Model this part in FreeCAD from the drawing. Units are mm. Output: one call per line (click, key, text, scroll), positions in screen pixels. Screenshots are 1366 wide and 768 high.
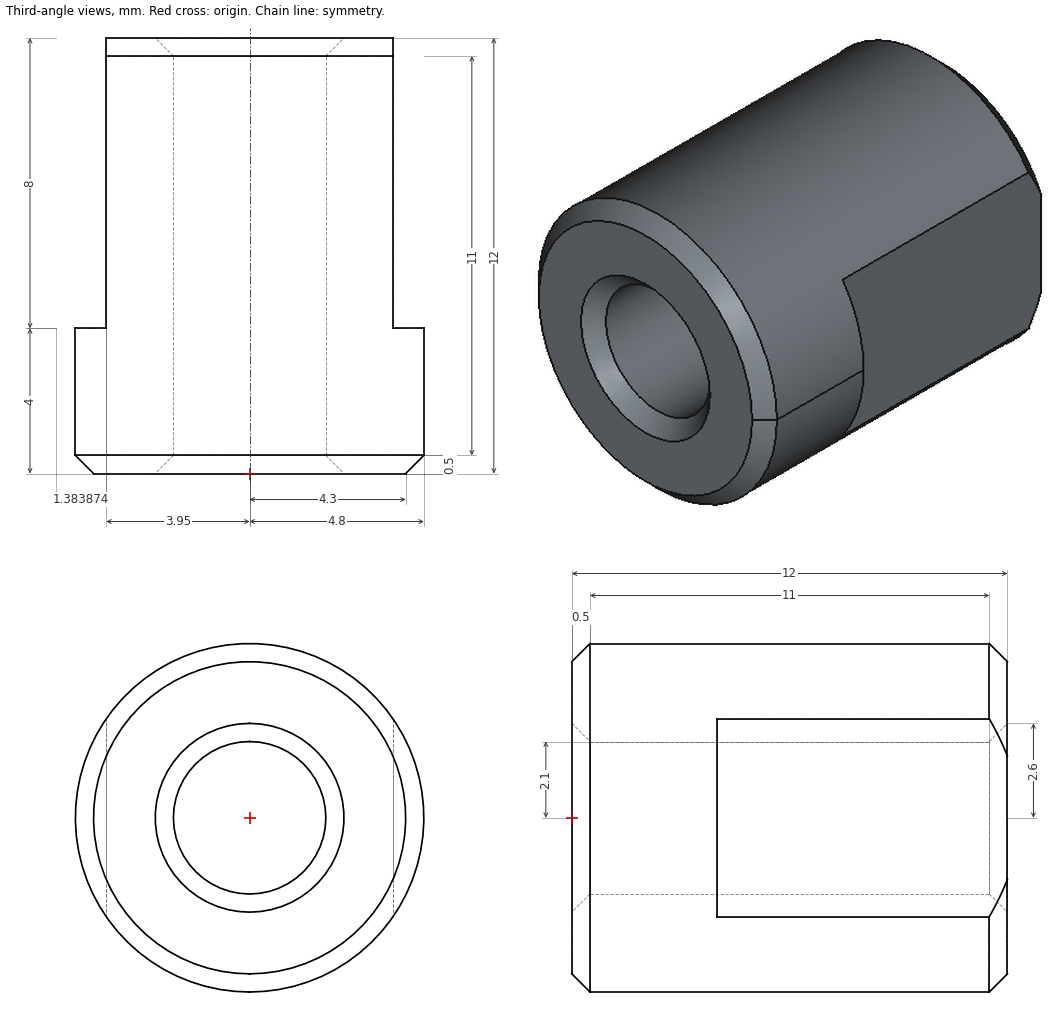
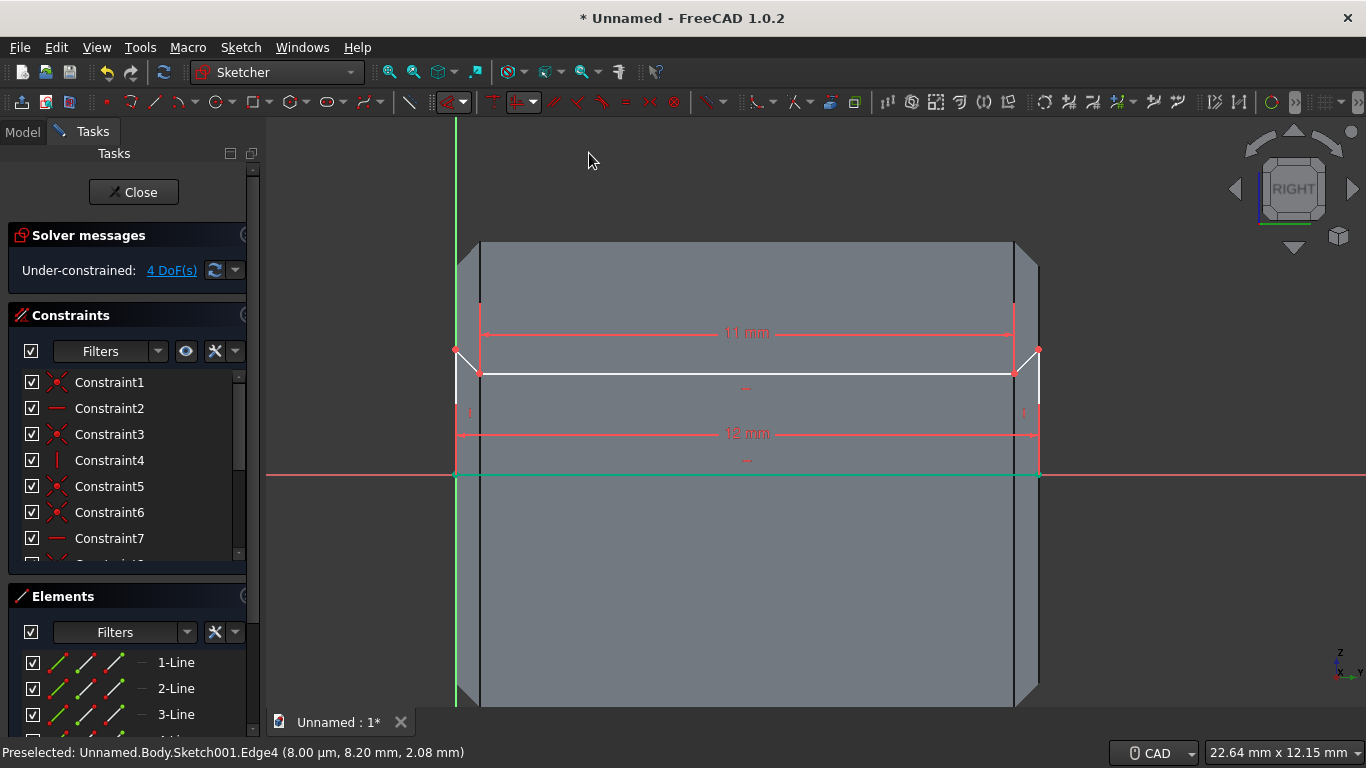
click(1039, 437)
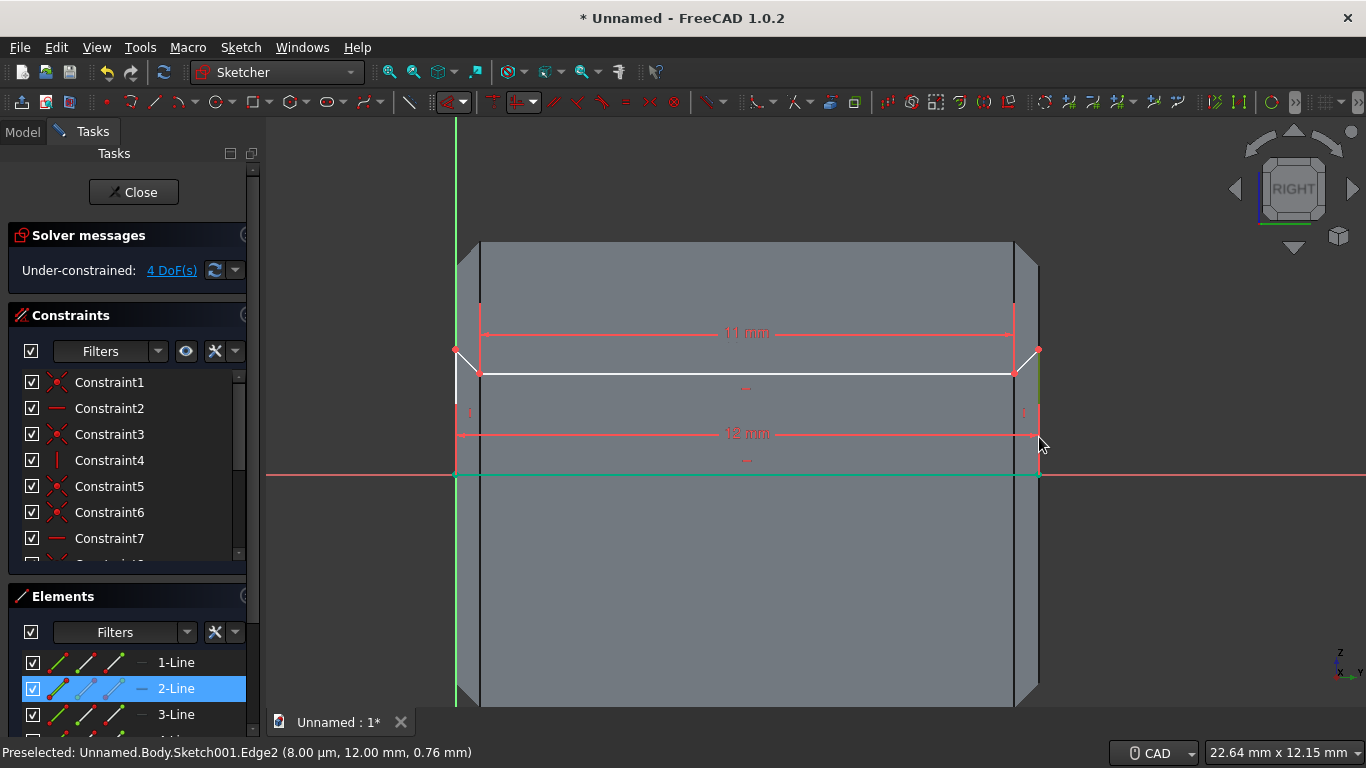
key(i)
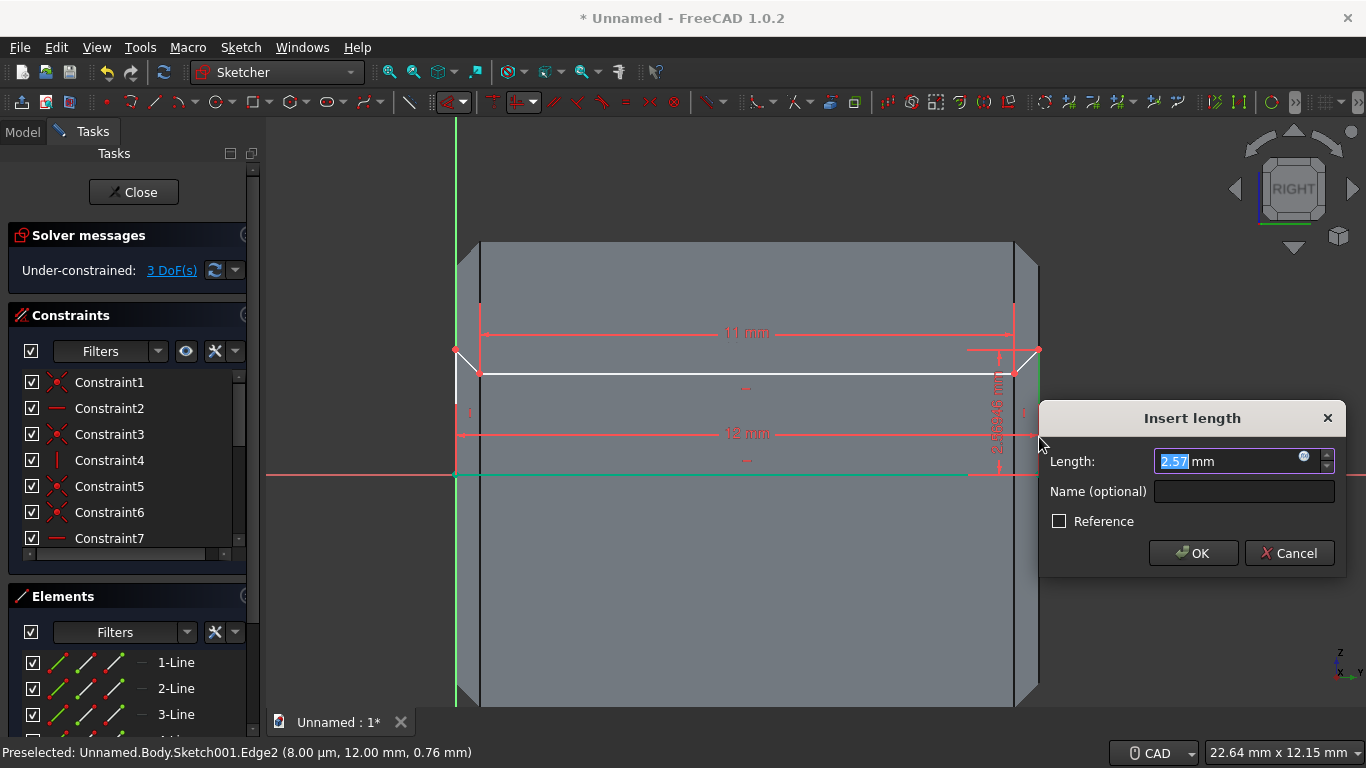
text(2.6)
key(Return)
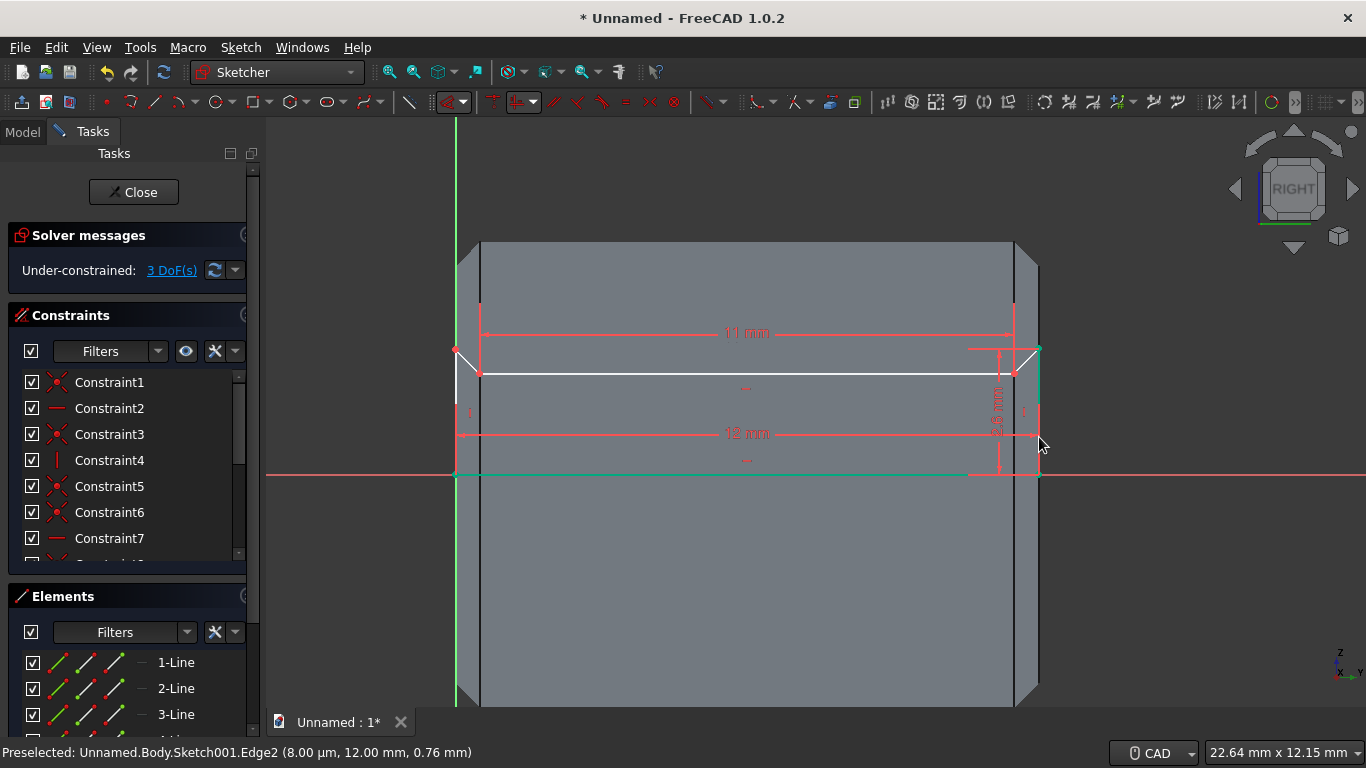
click(456, 387)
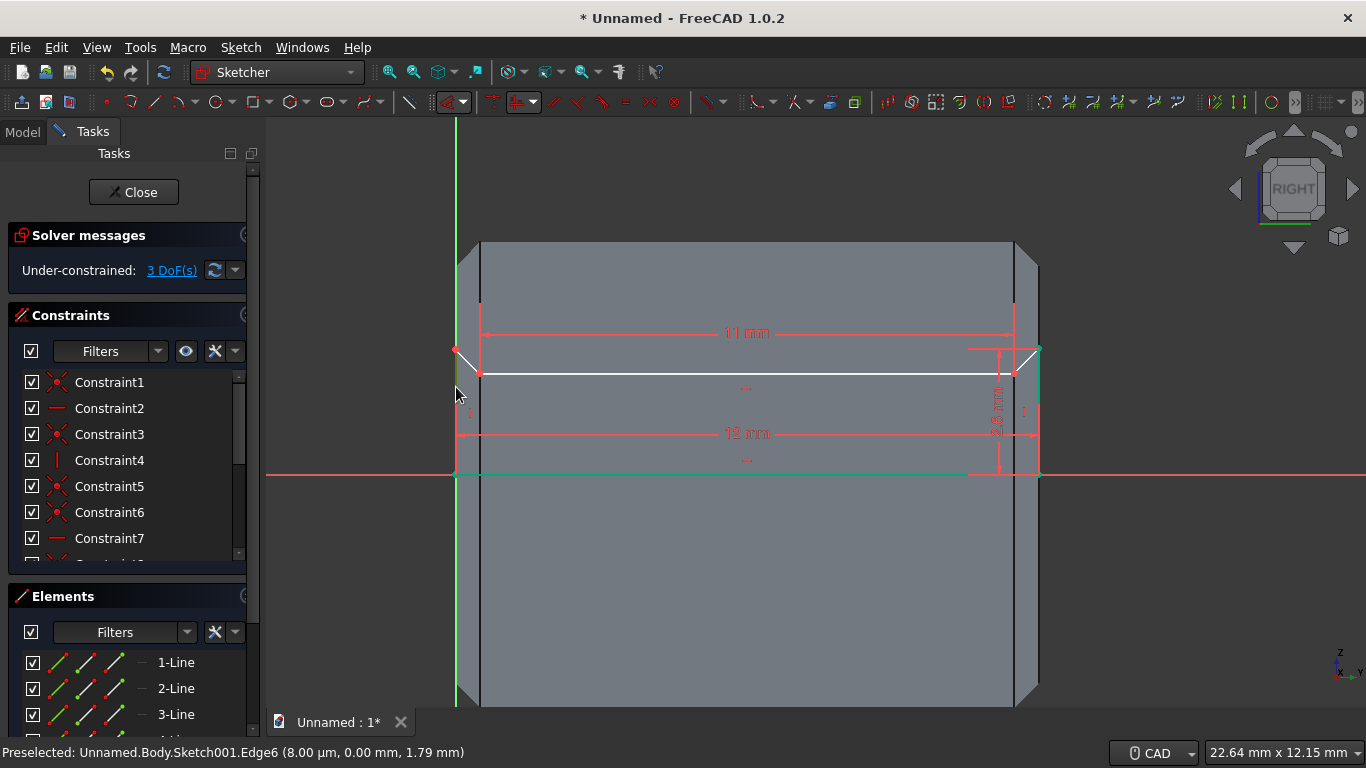
click(466, 102)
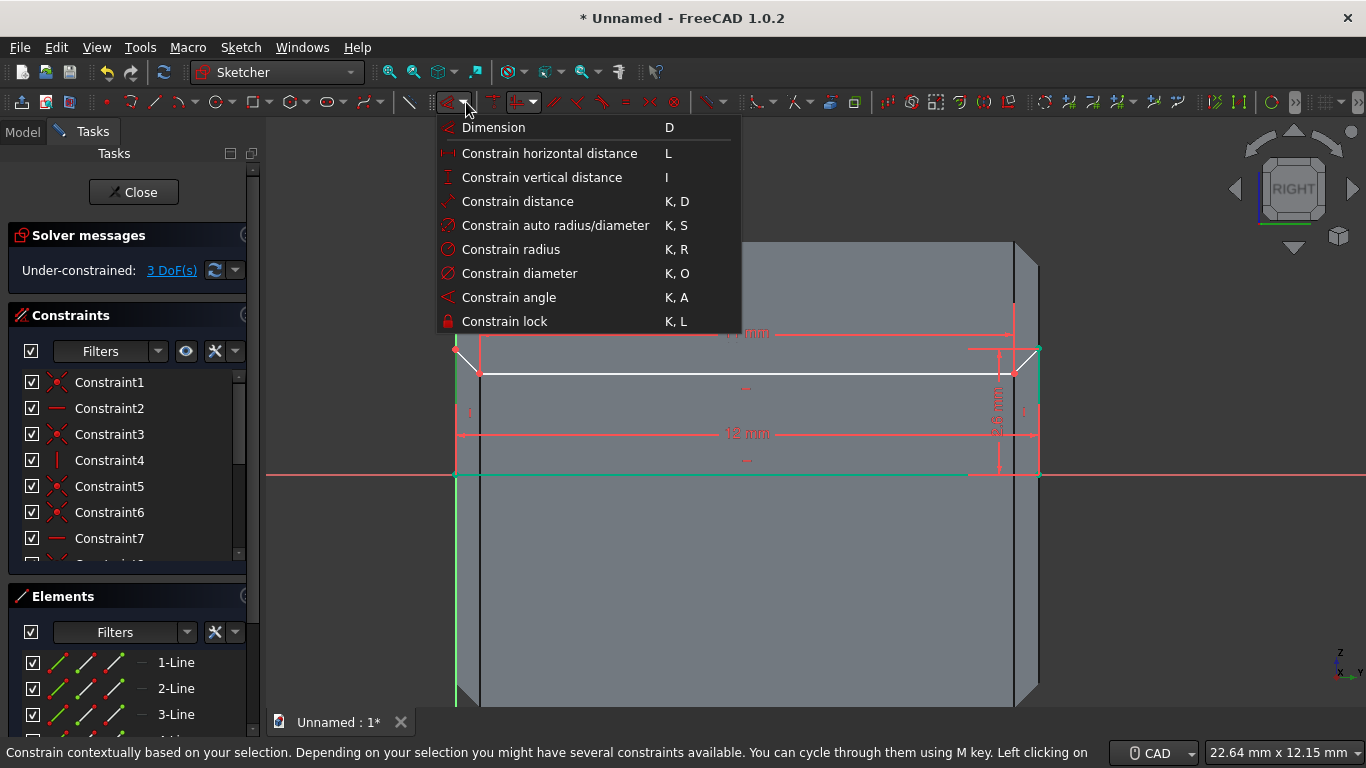
click(589, 177)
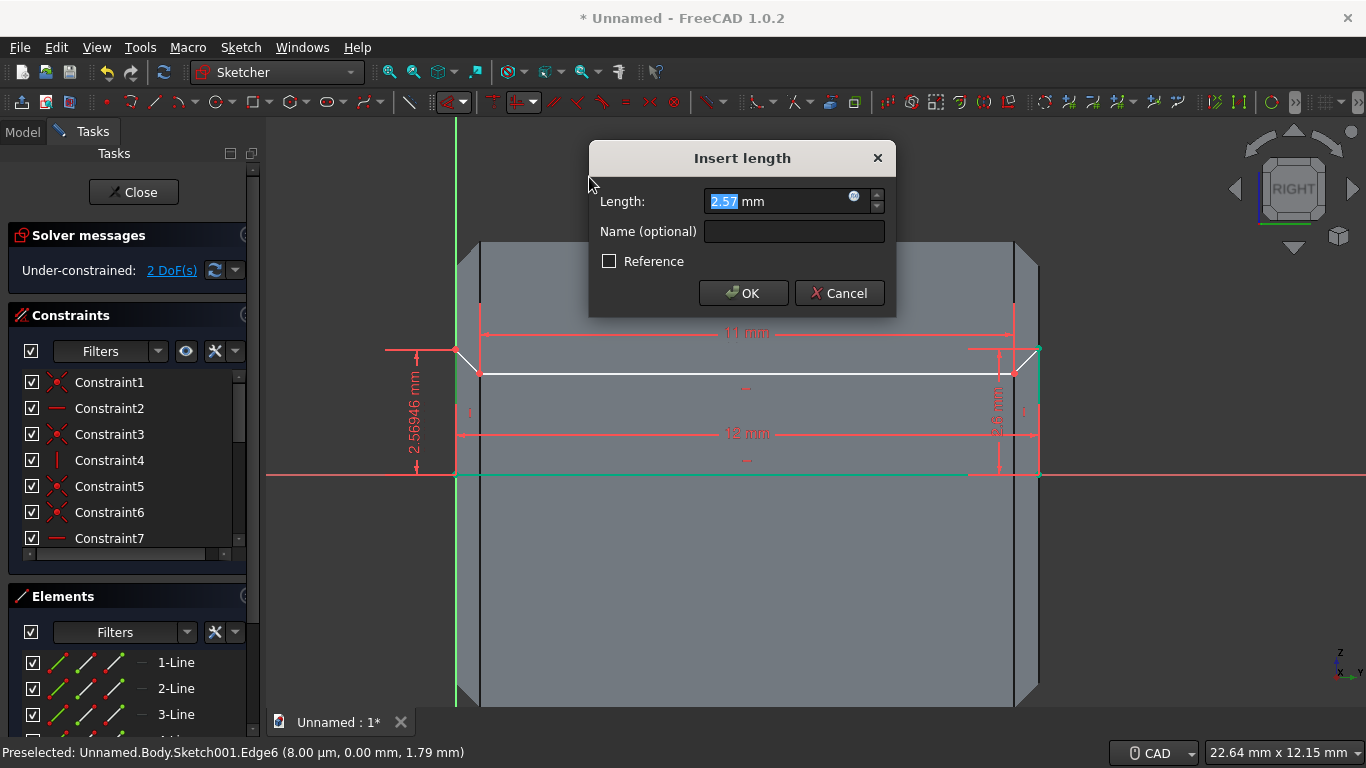
text(2.6)
key(Return)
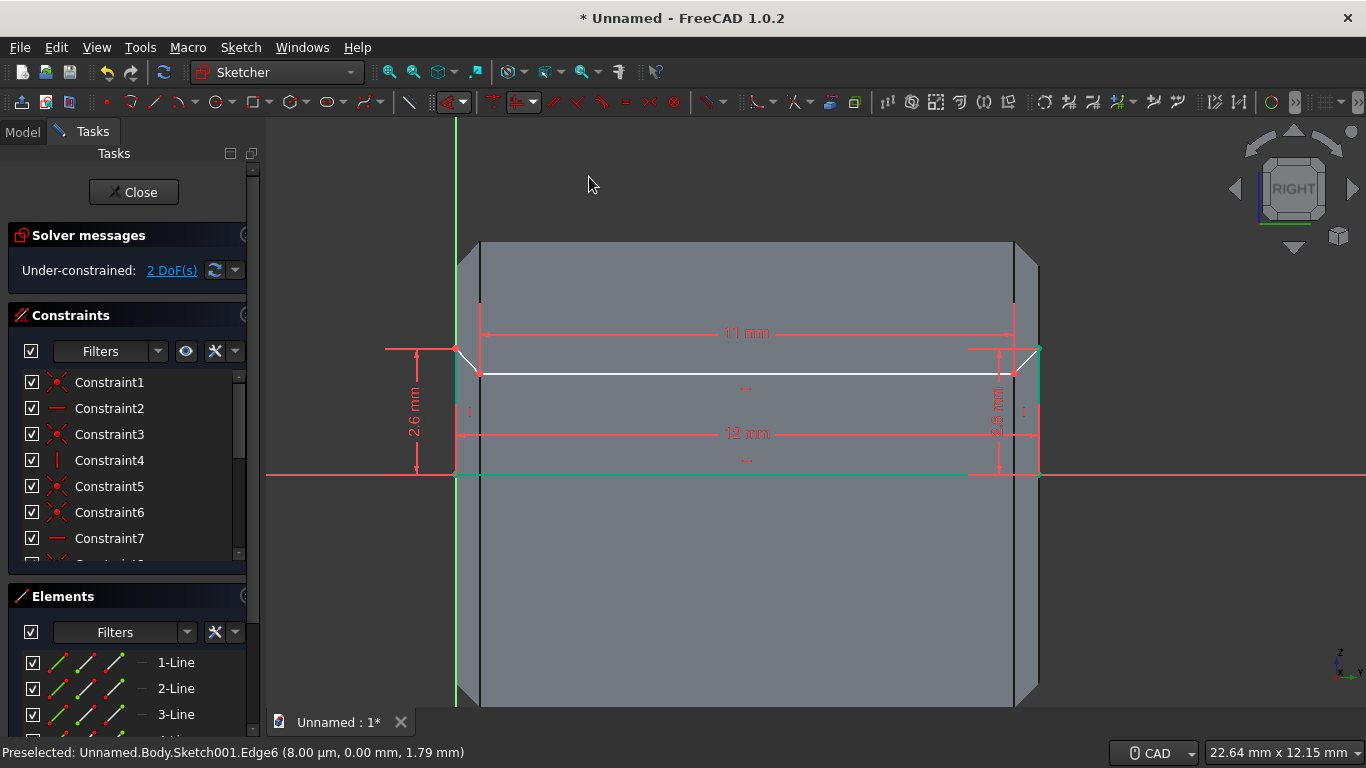
click(1014, 374)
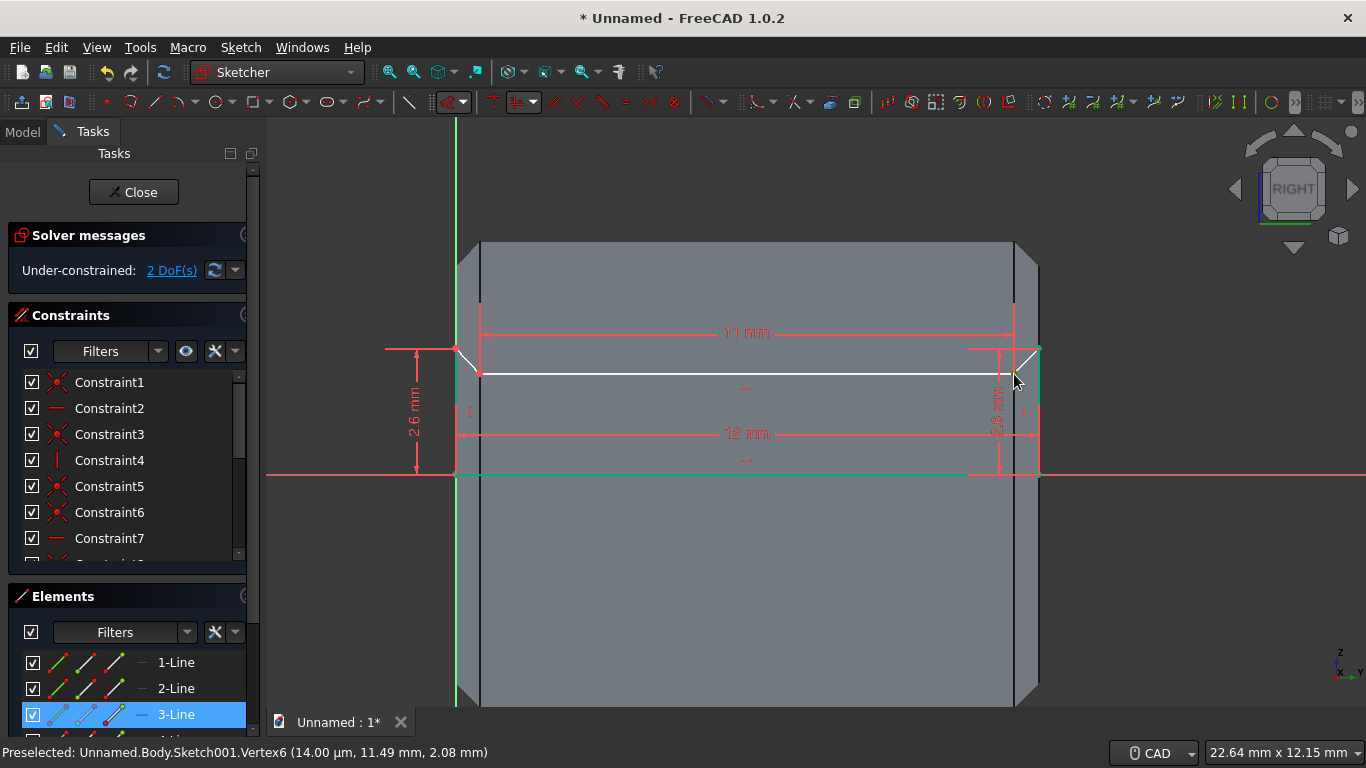
key(i)